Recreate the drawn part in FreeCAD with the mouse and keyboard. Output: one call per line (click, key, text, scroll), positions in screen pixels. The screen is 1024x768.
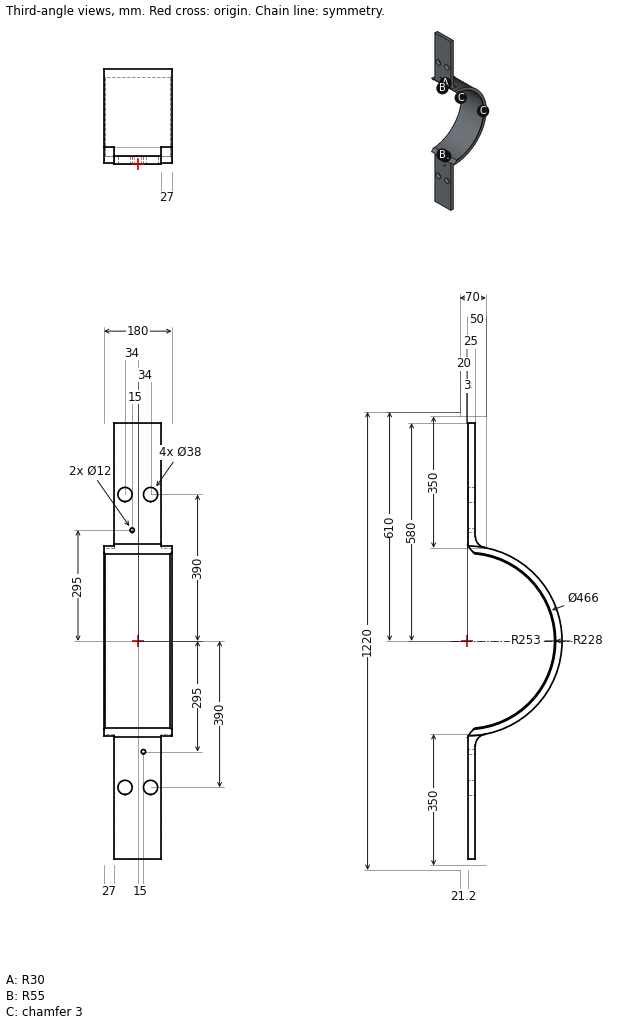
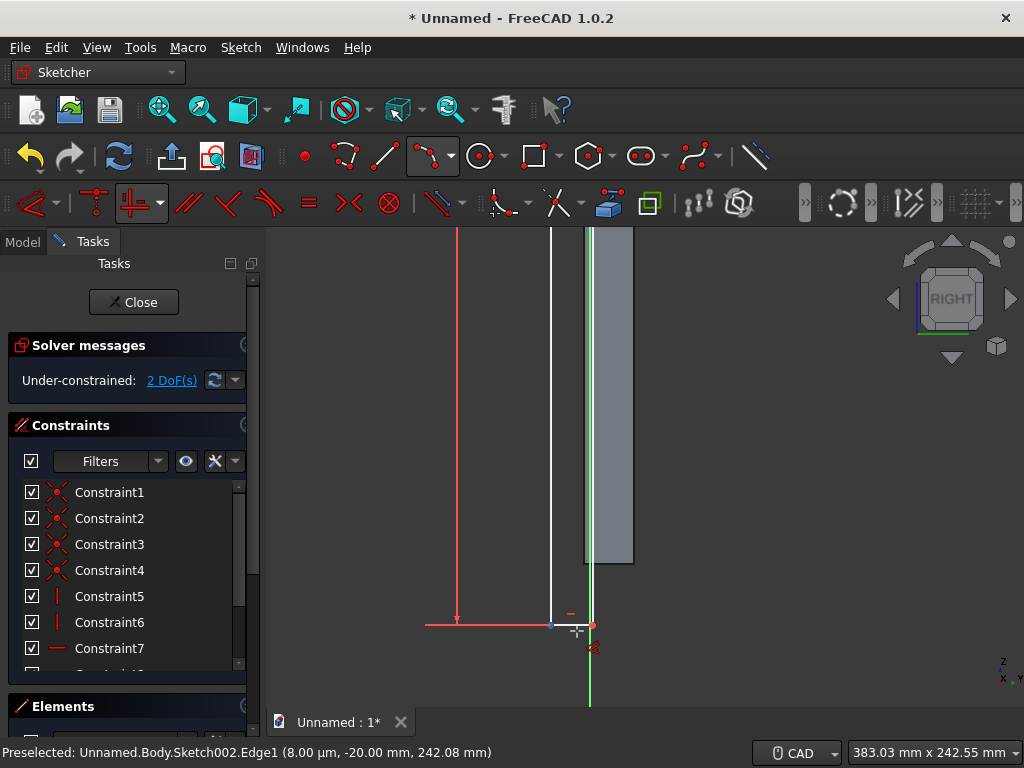
click(572, 625)
click(572, 659)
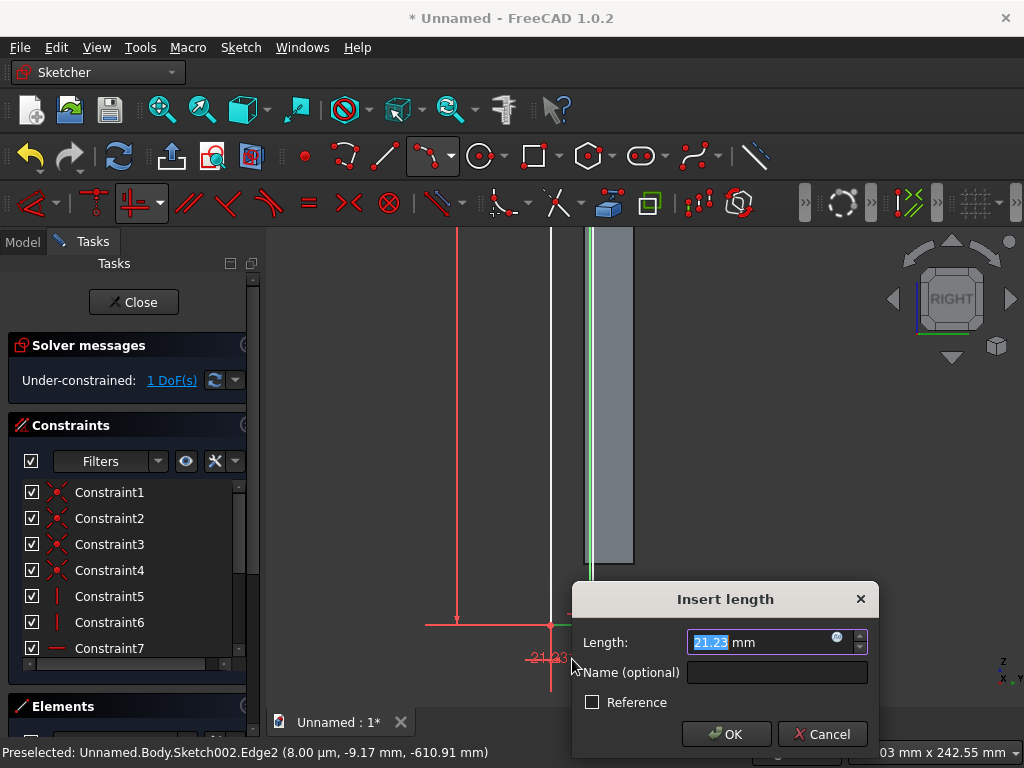
text(21.2)
key(Return)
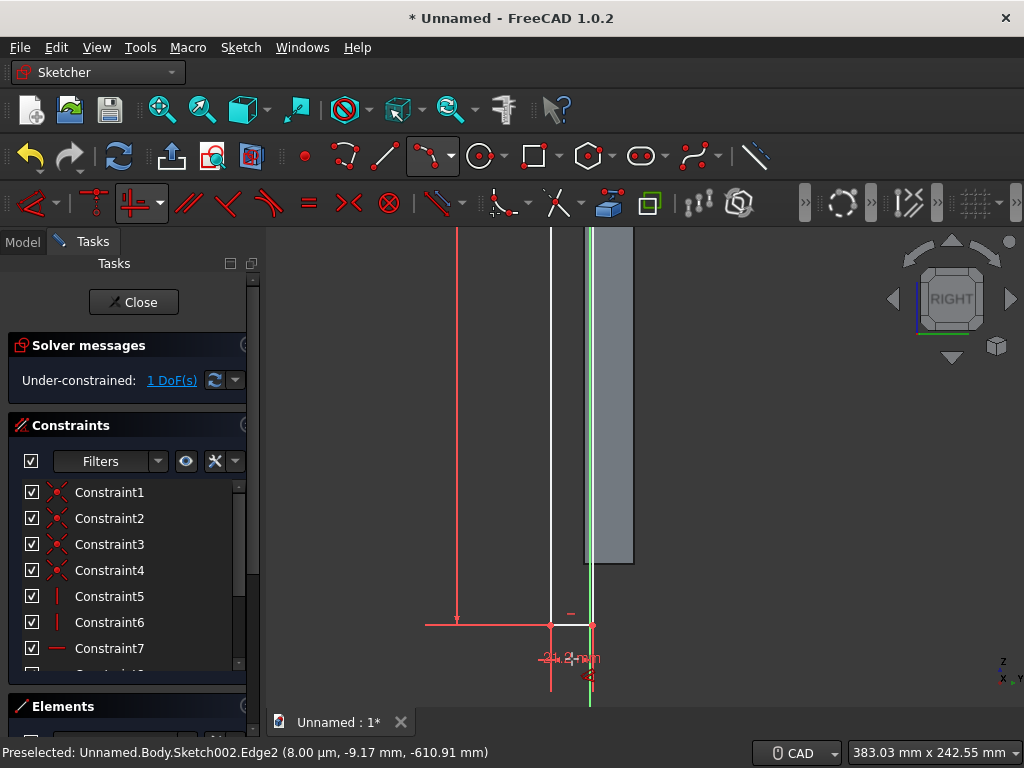
scroll(577, 631, down, 10)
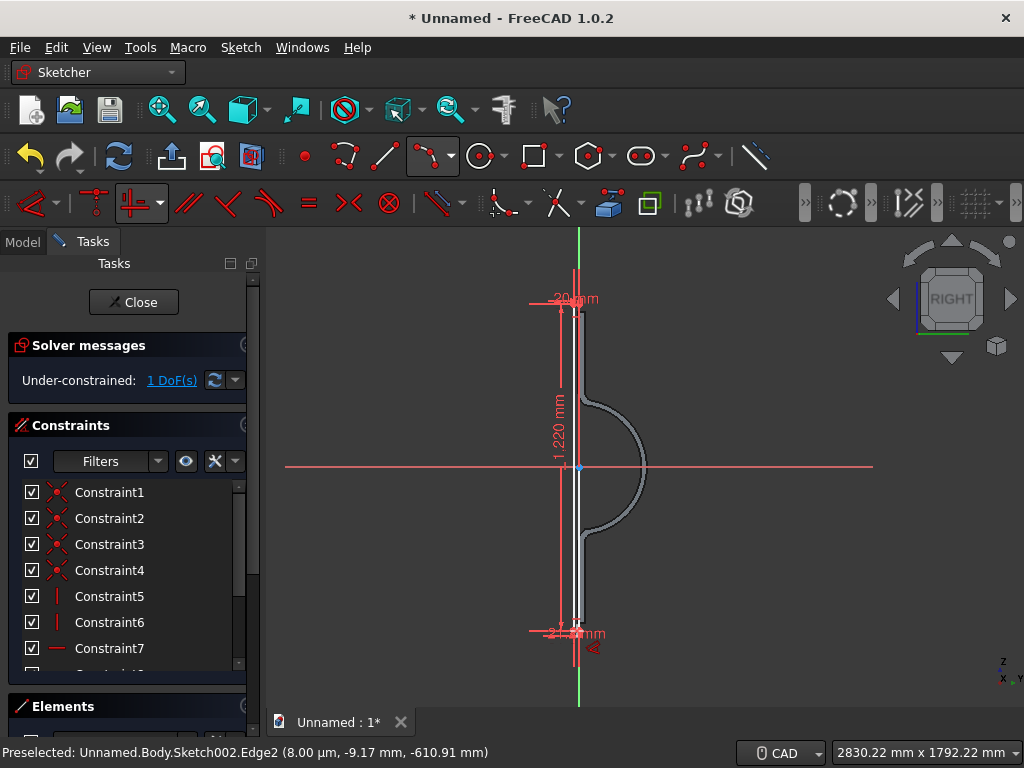
scroll(574, 304, up, 4)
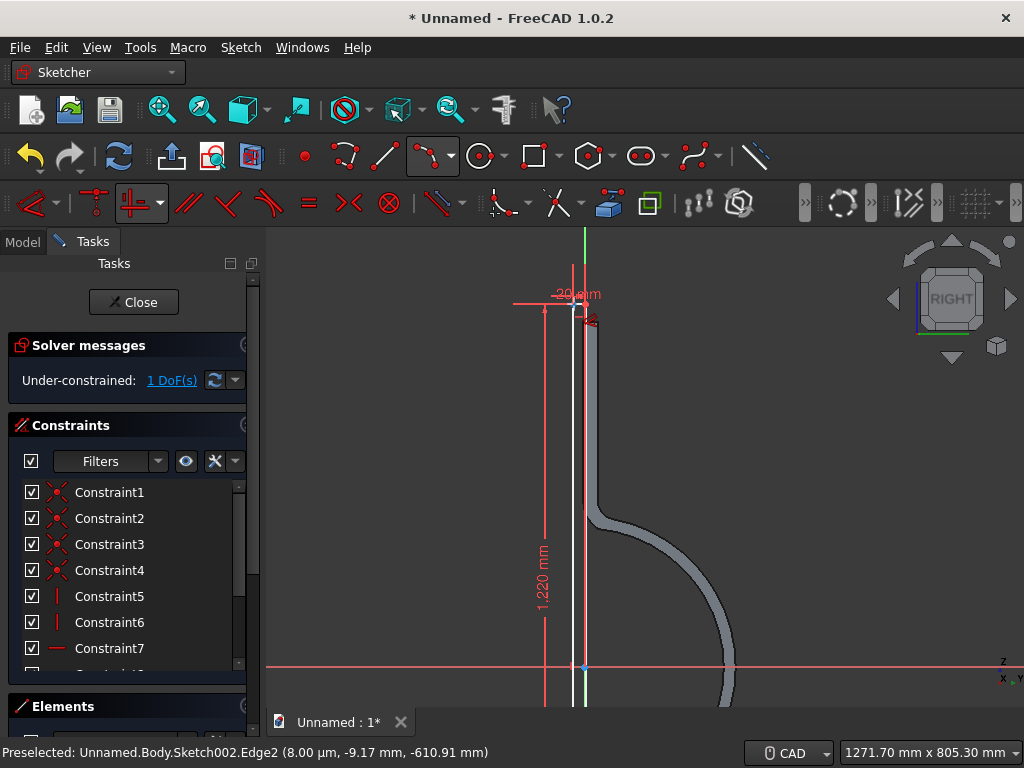
click(573, 304)
click(539, 486)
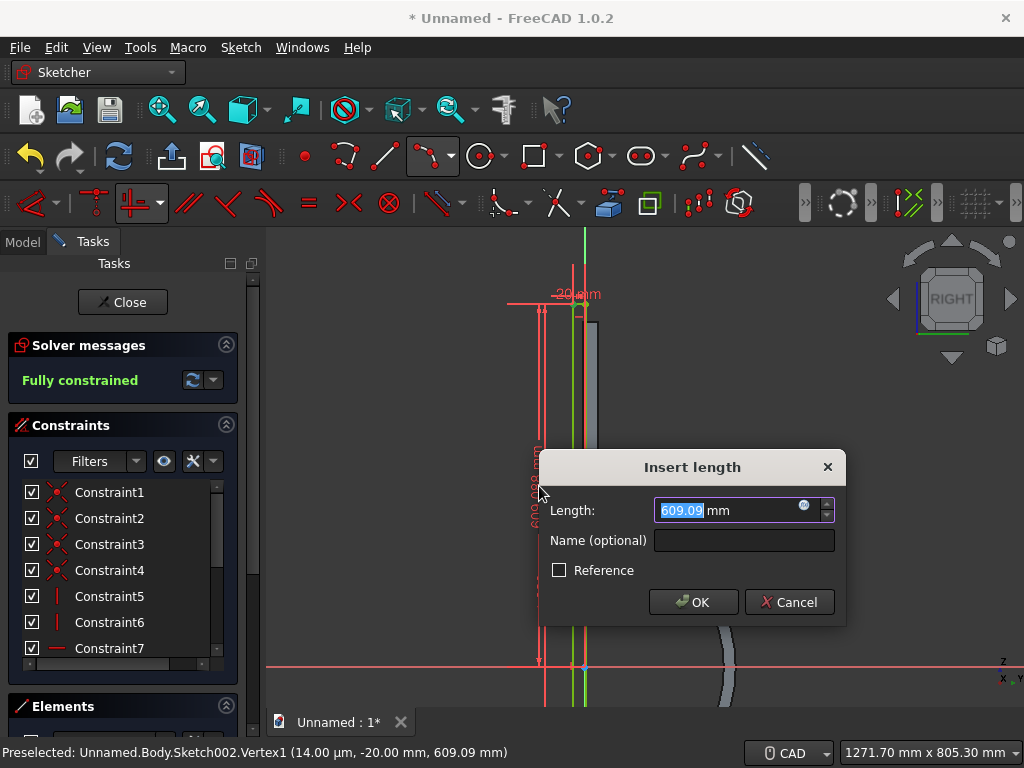
text(610)
key(Return)
key(Escape)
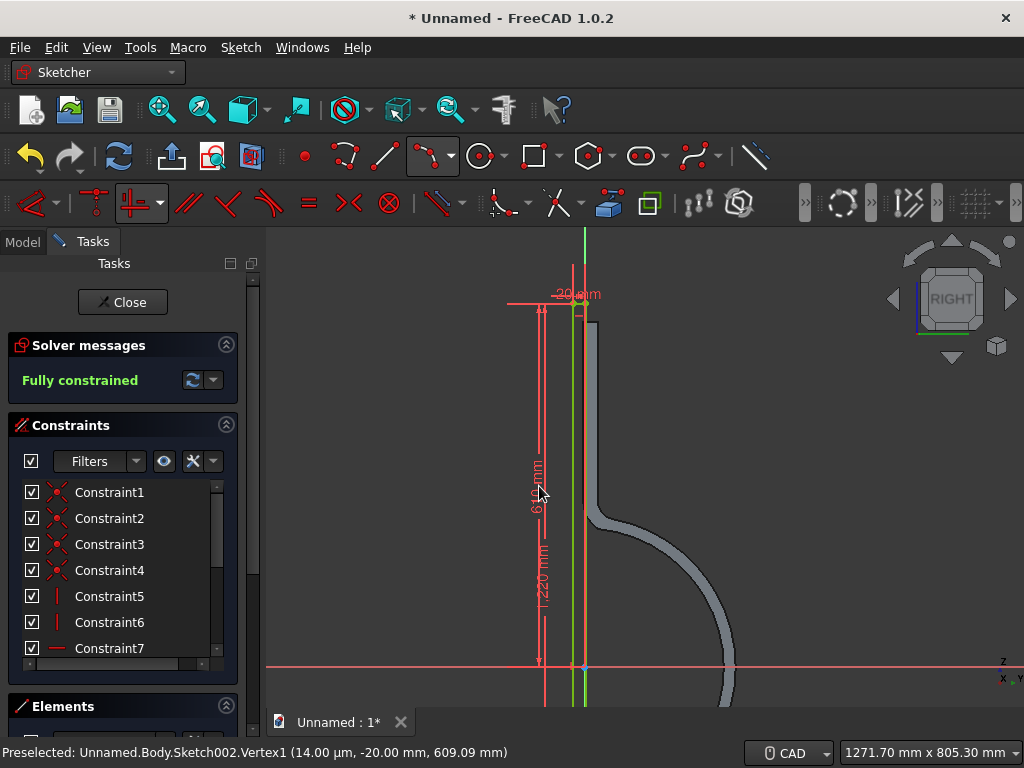
click(123, 302)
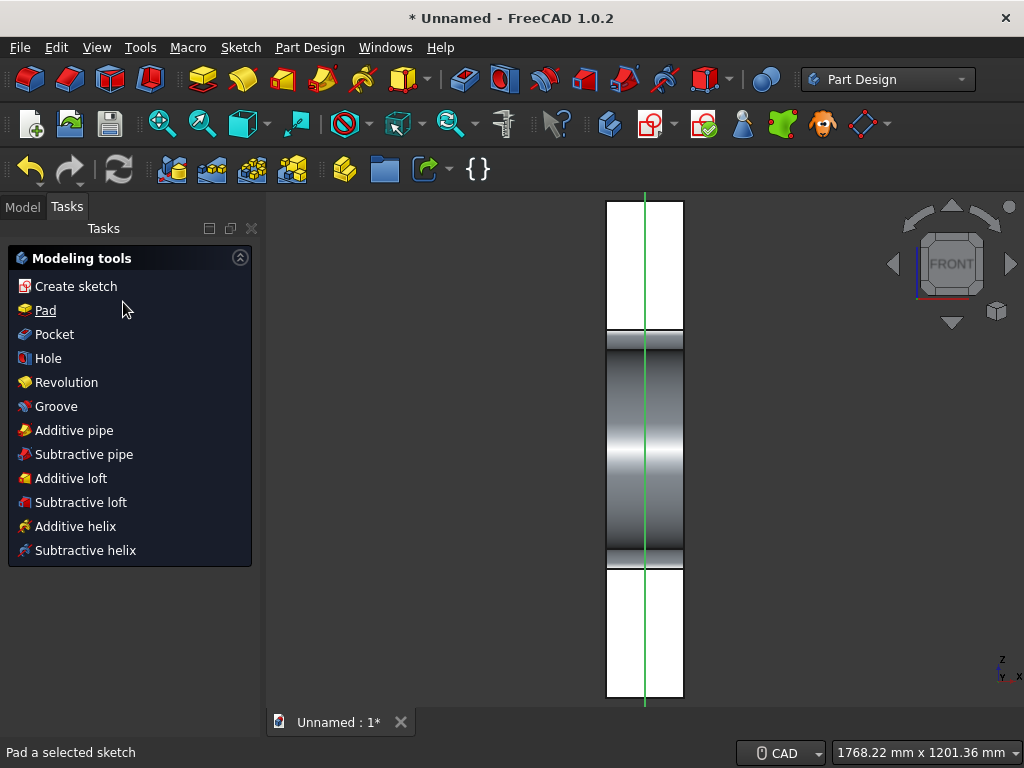
click(466, 80)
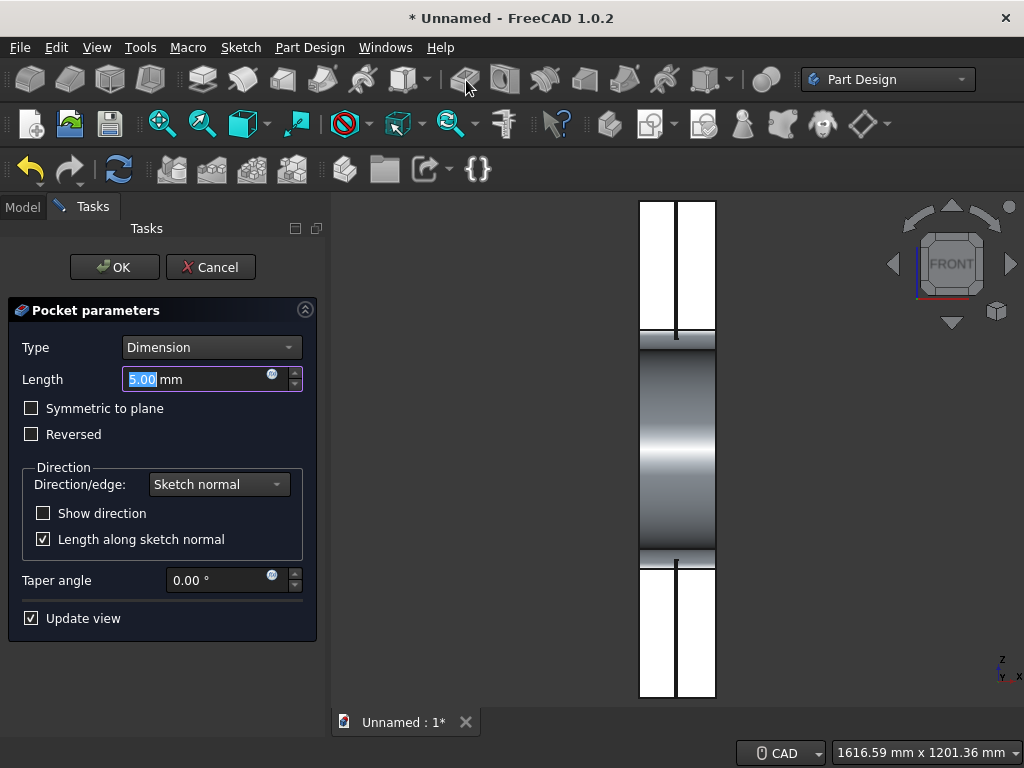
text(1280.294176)
key(Tab)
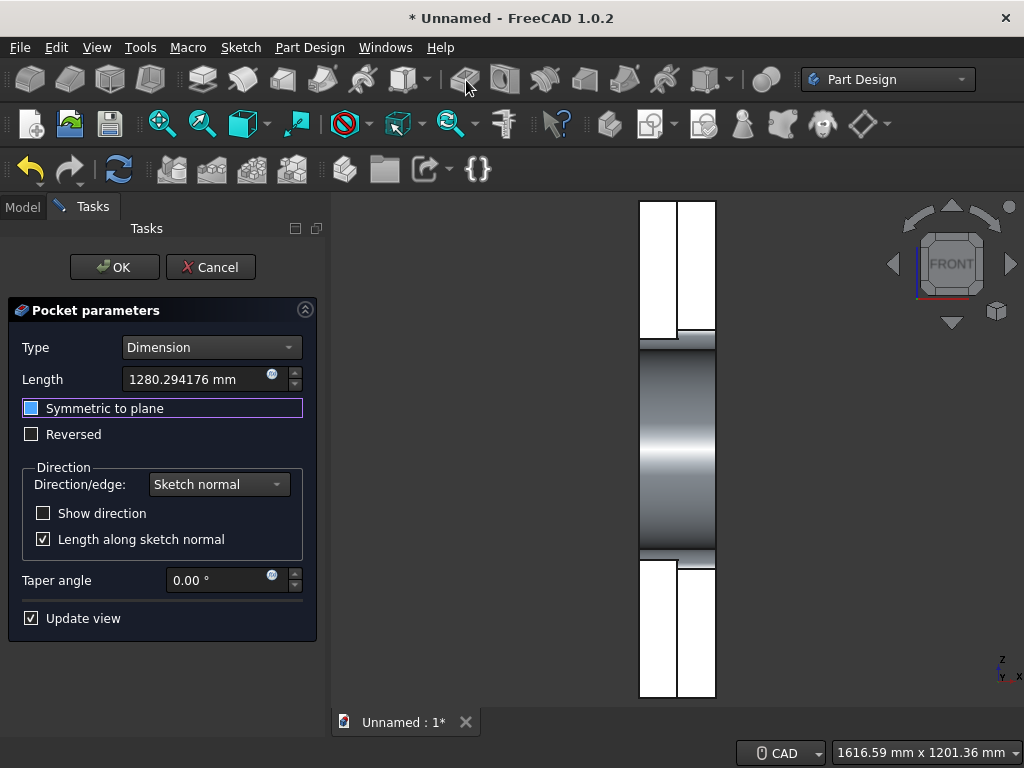
click(30, 408)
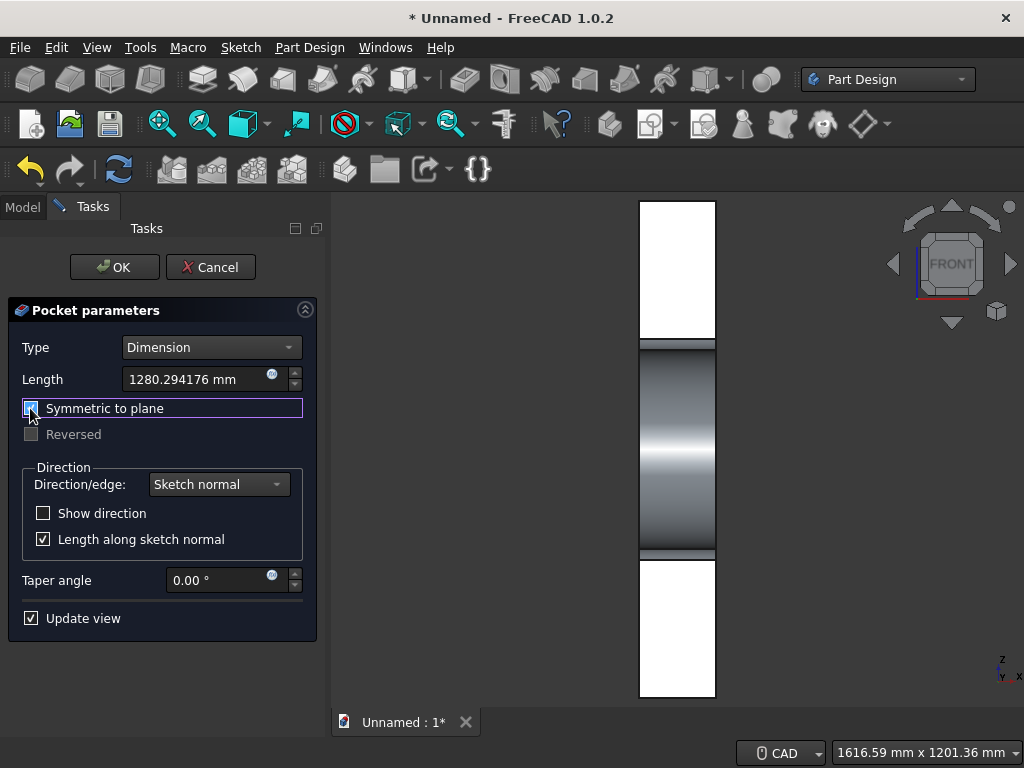
click(115, 267)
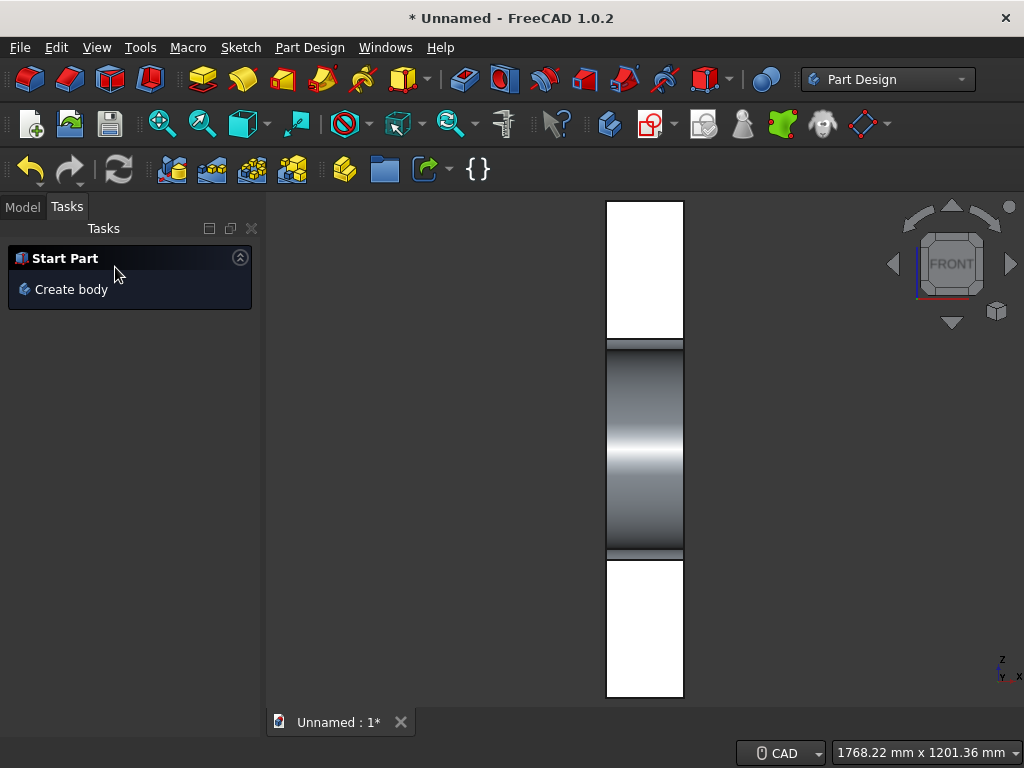
key(0)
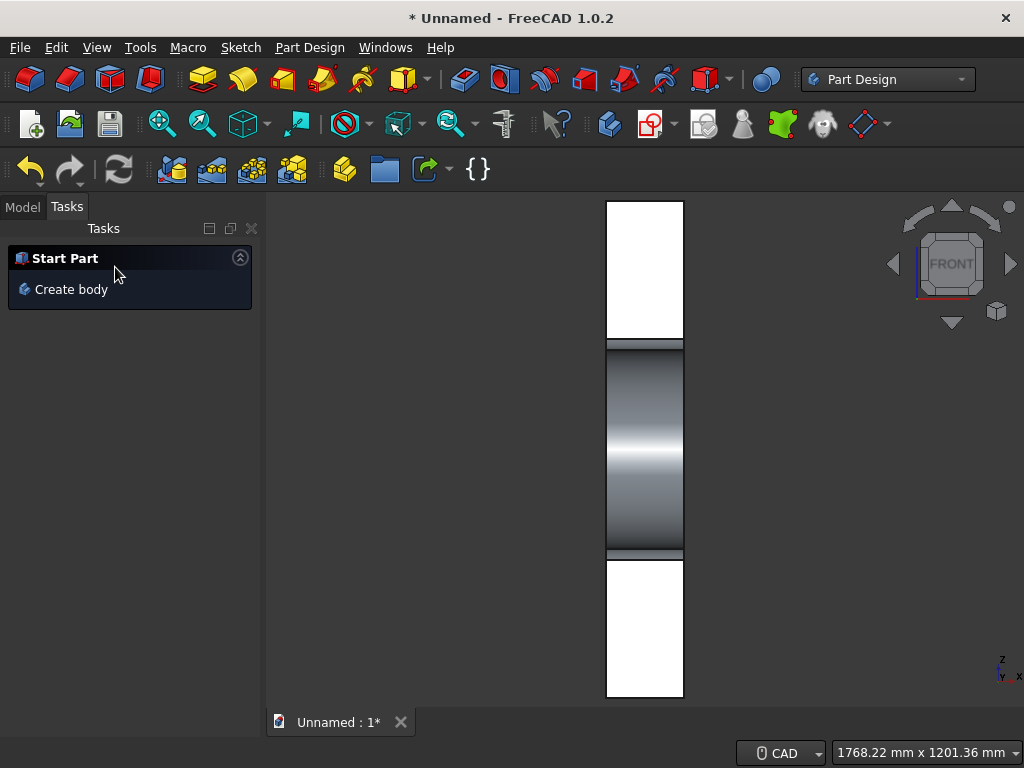
scroll(640, 657, up, 12)